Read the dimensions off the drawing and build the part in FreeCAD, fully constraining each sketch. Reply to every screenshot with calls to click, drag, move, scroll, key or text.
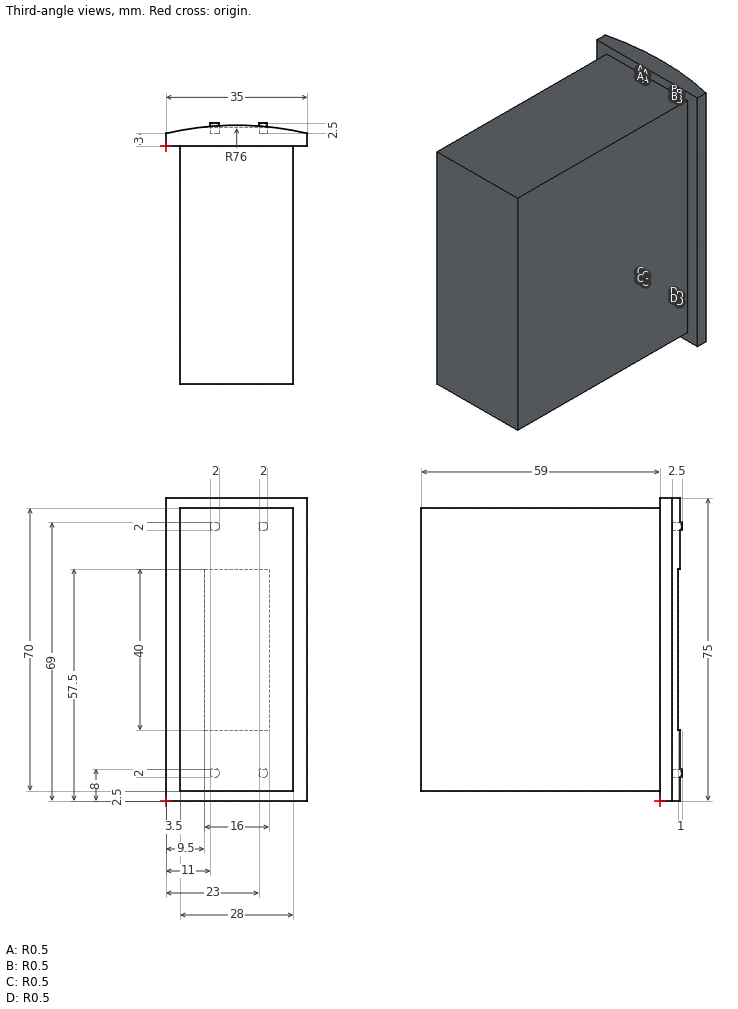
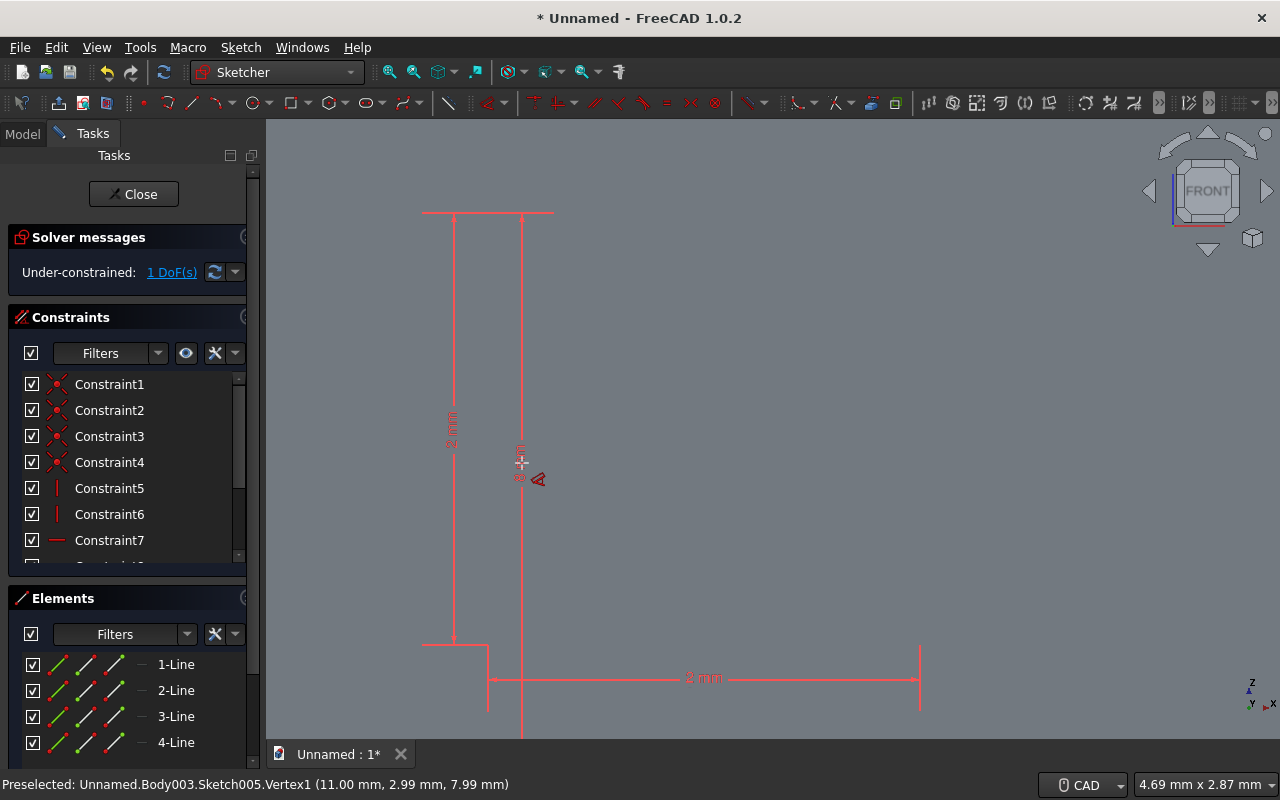
click(488, 213)
click(391, 179)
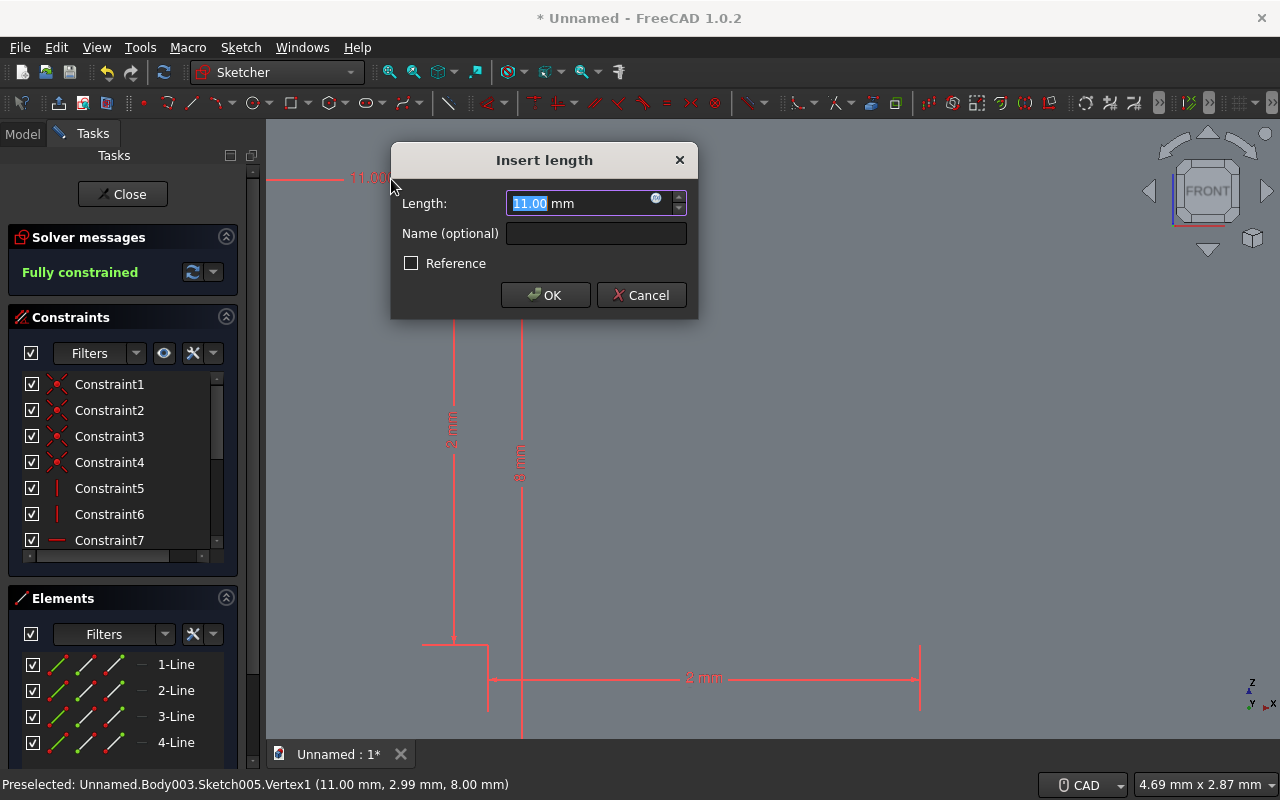
text(11)
key(Return)
key(Escape)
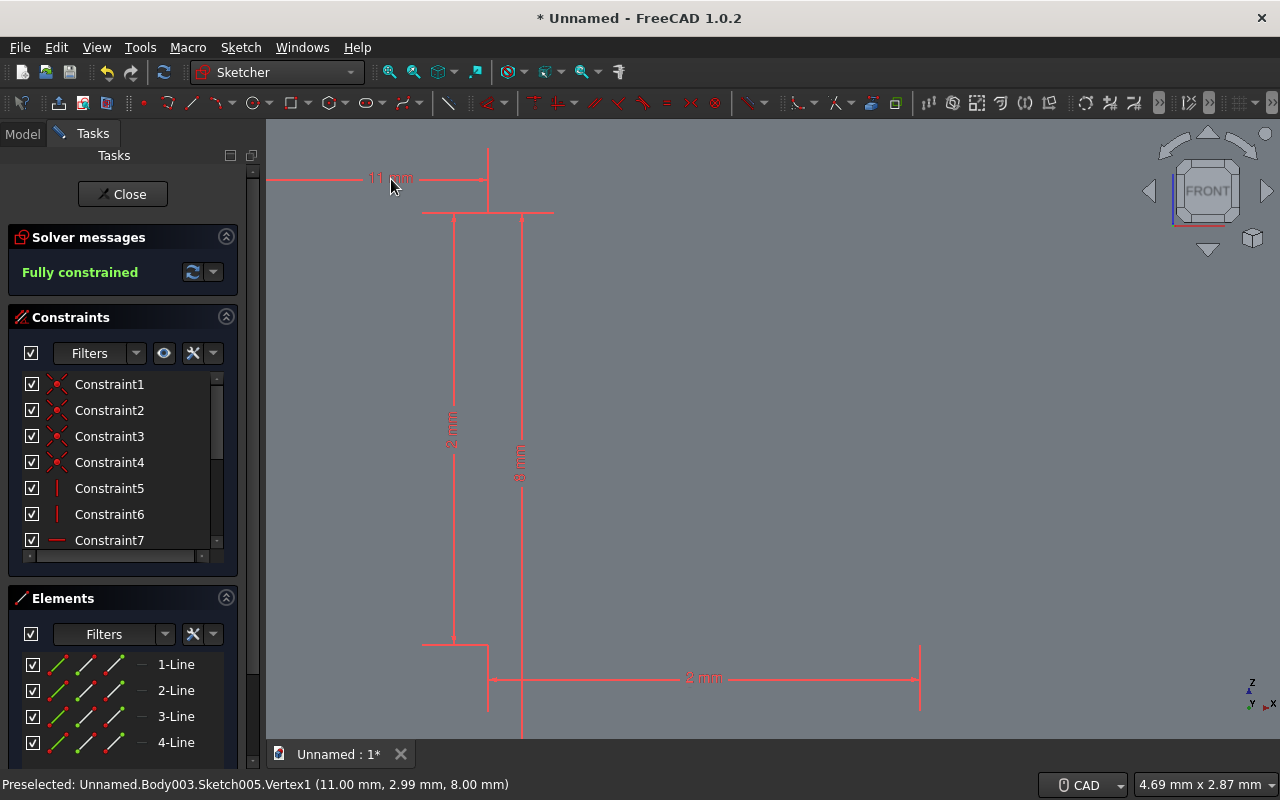
click(123, 194)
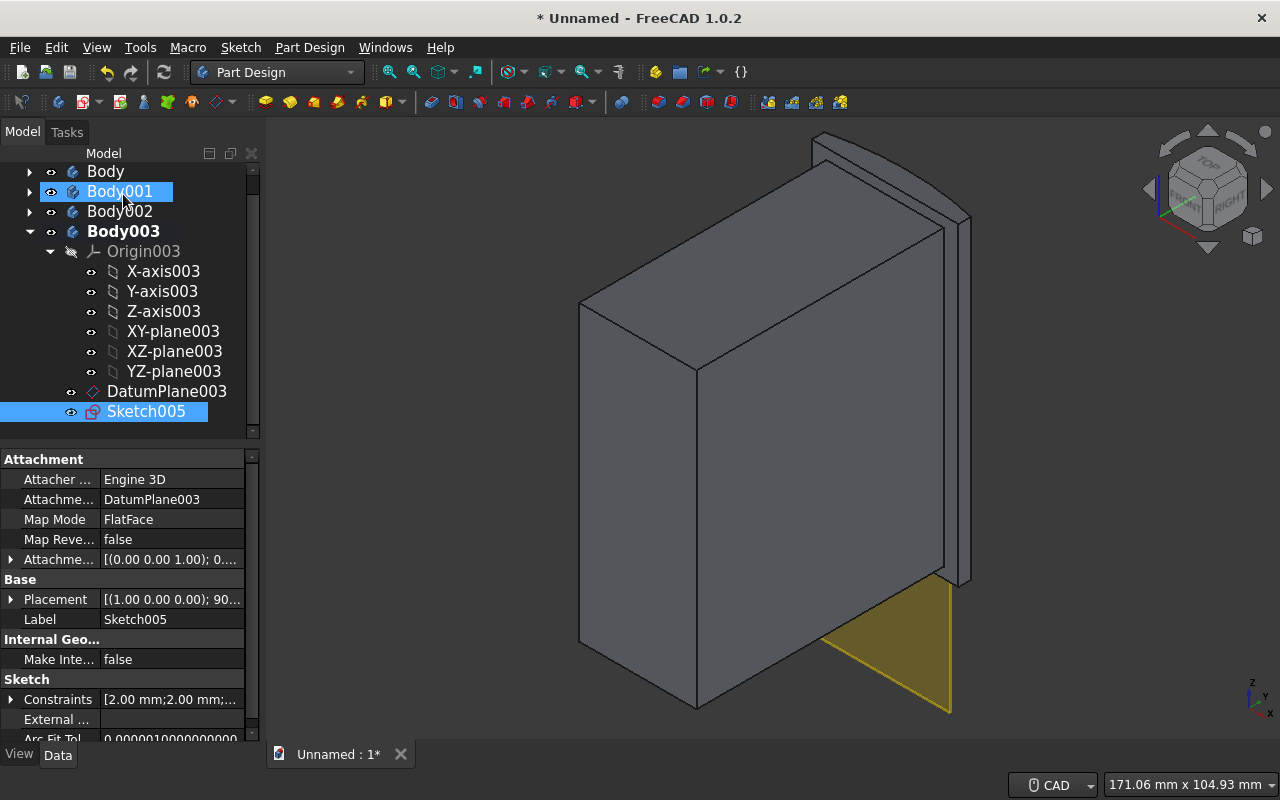
click(266, 102)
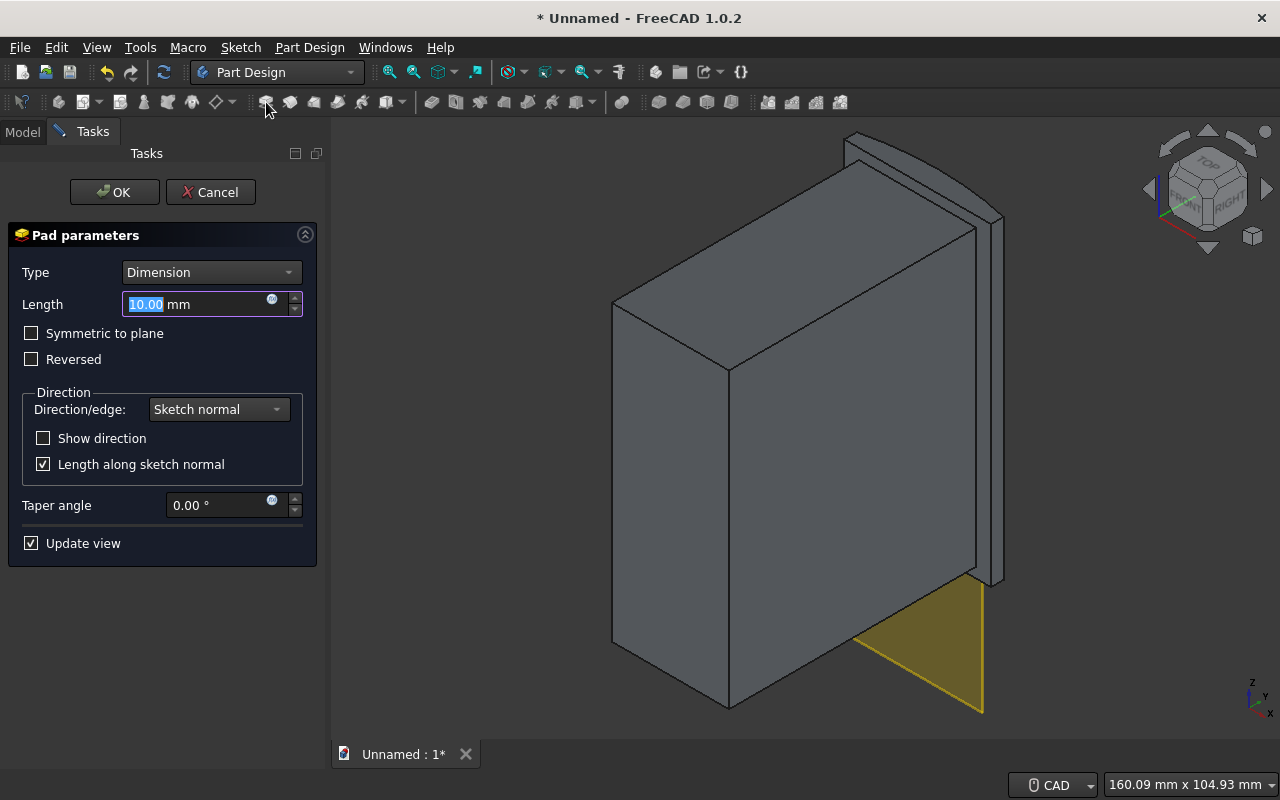
text(2.5)
key(Tab)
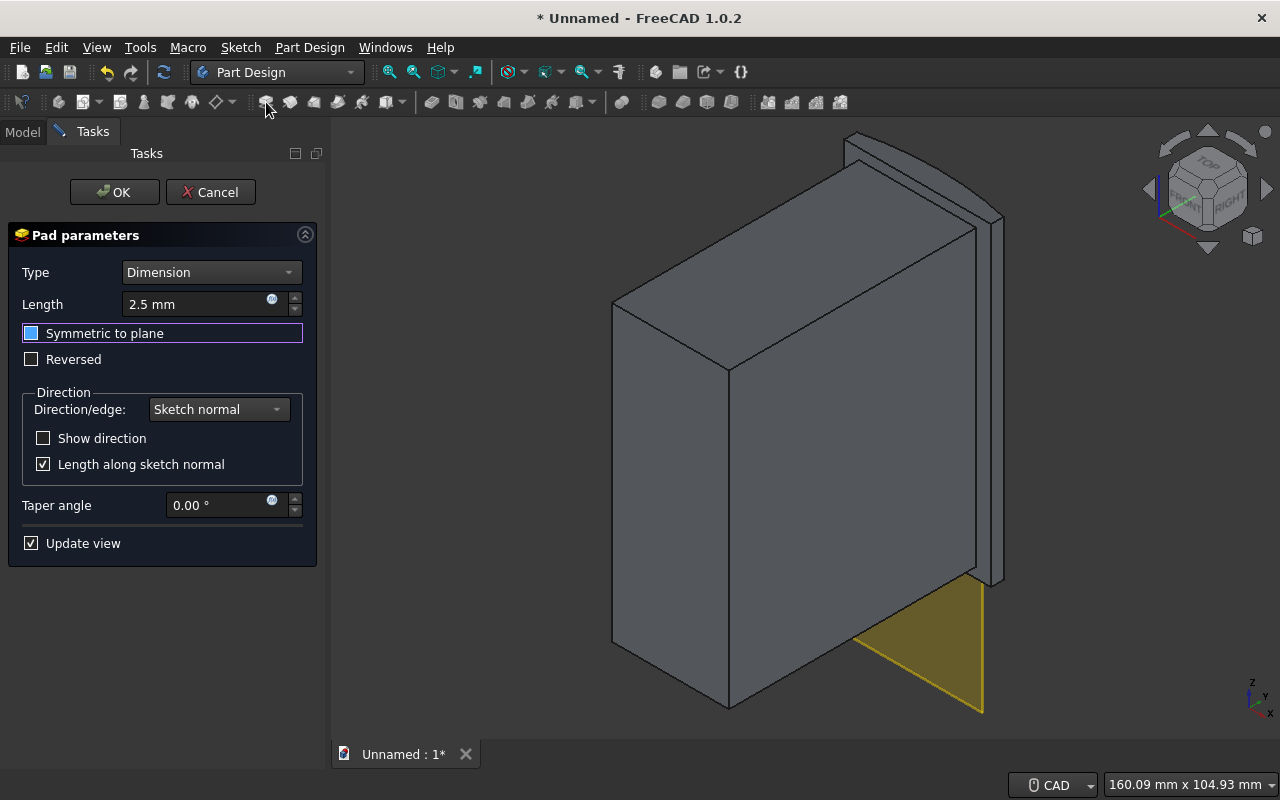
click(30, 359)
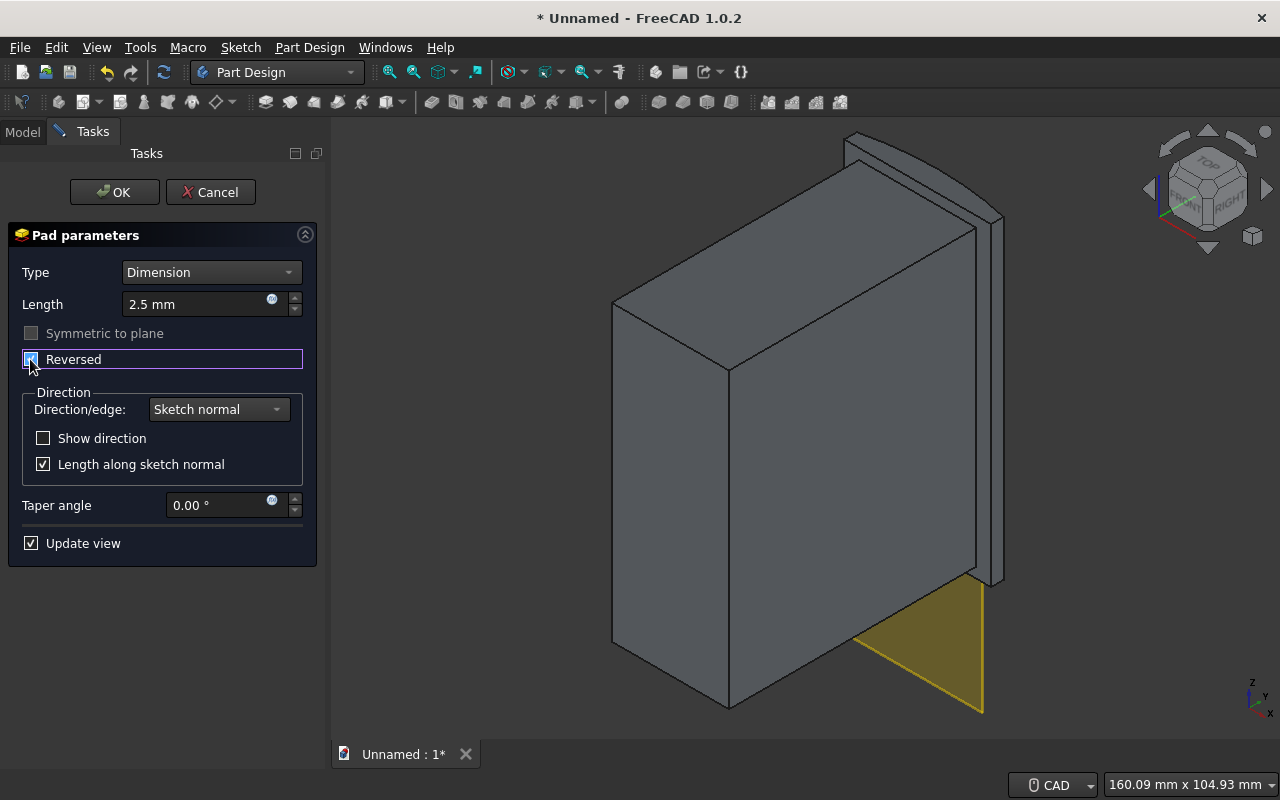
click(115, 192)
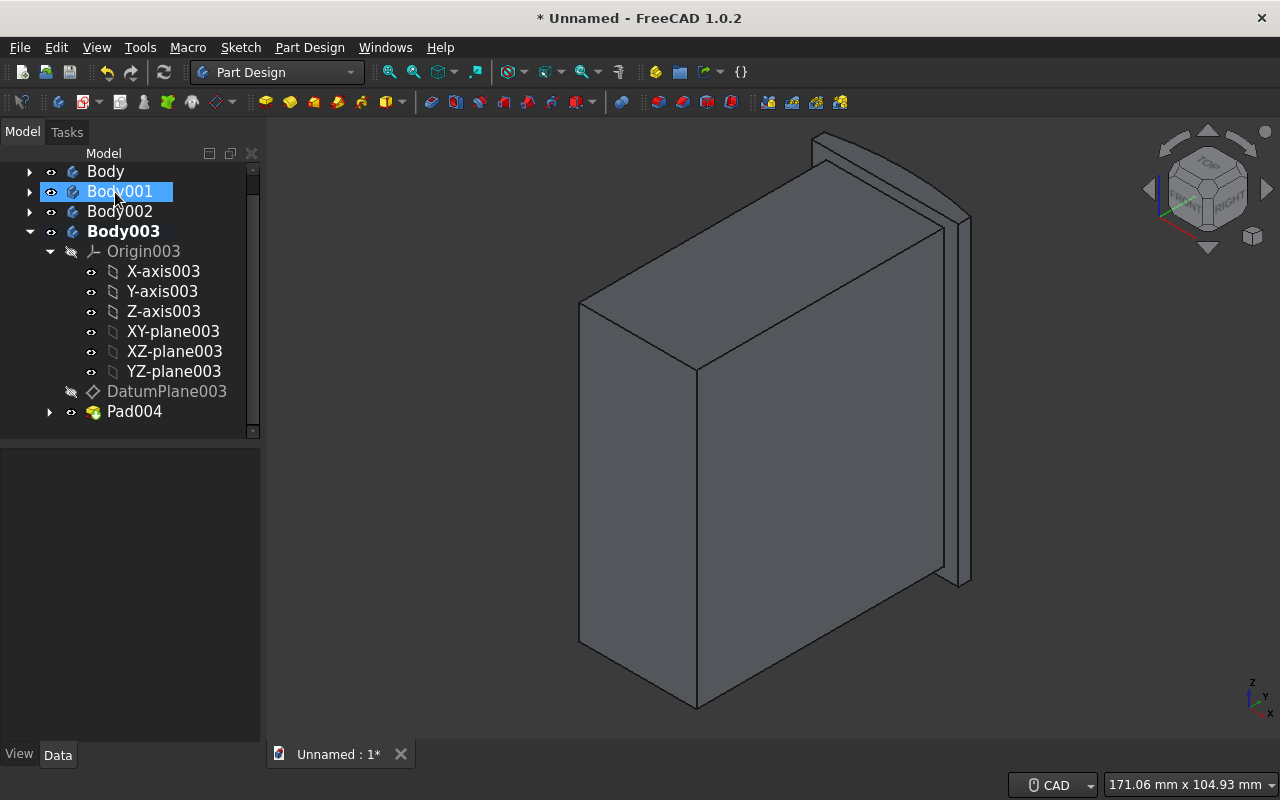
key(v)
key(f)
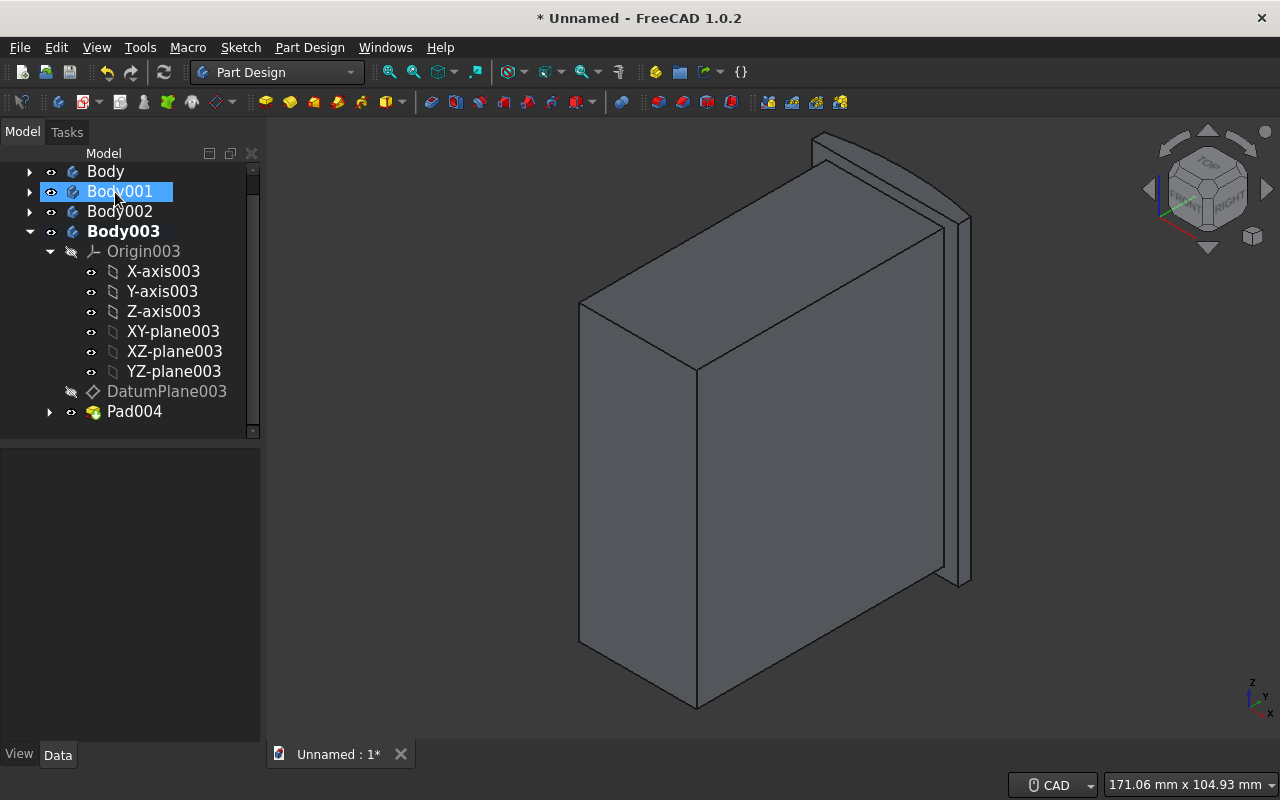
scroll(876, 479, up, 5)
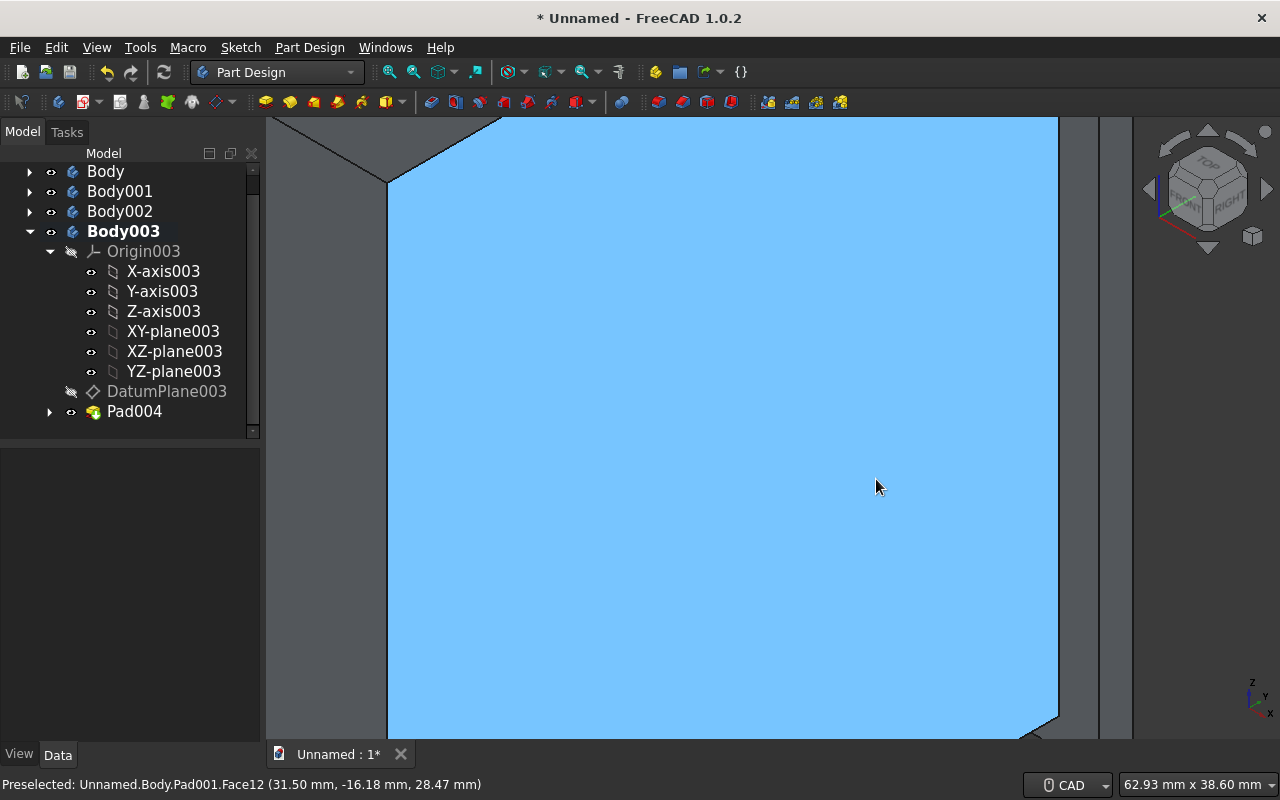
key(v)
key(f)